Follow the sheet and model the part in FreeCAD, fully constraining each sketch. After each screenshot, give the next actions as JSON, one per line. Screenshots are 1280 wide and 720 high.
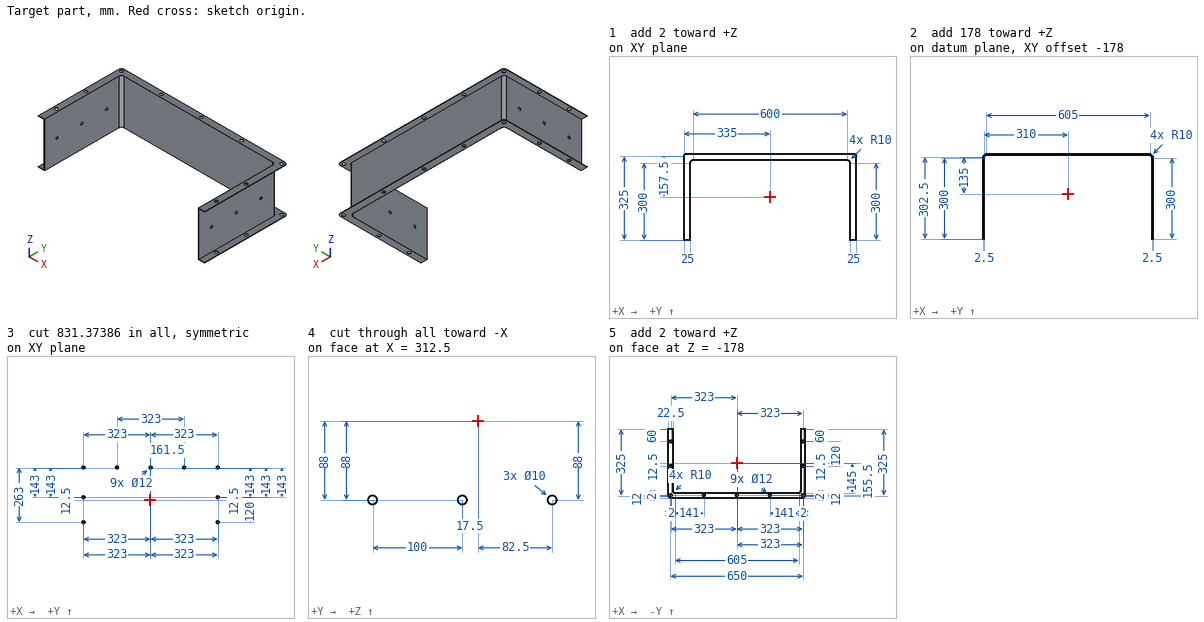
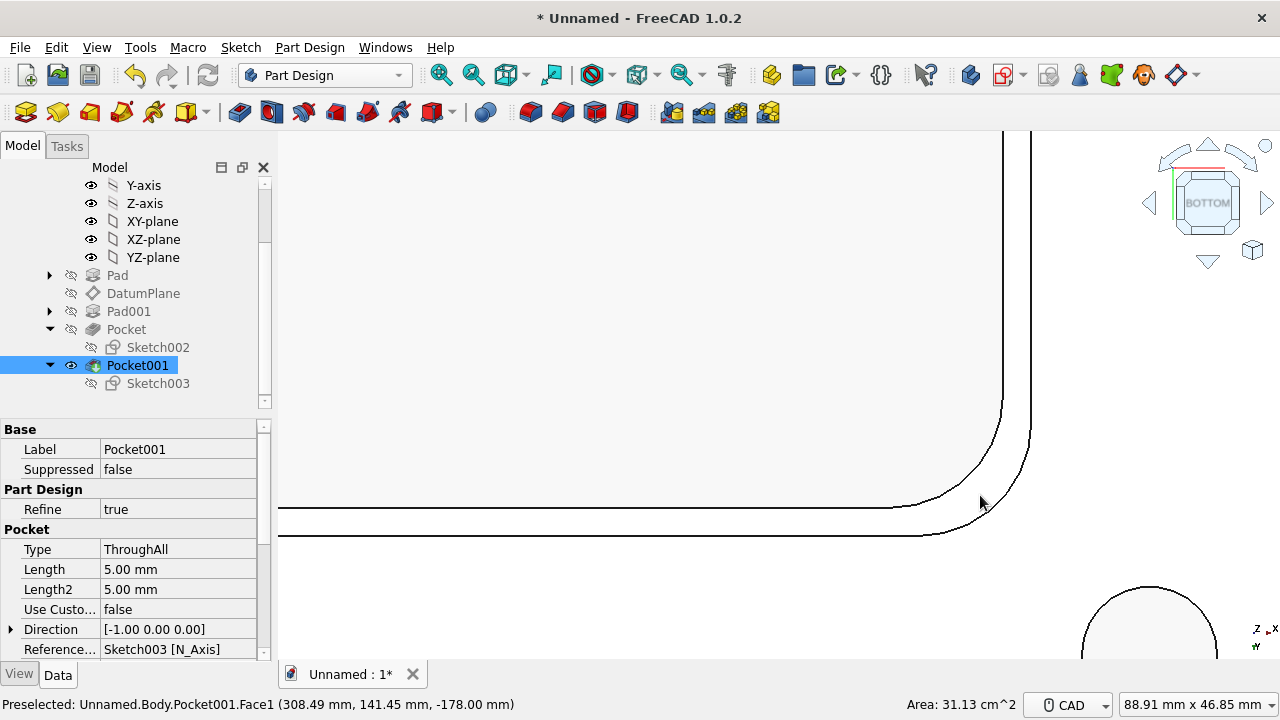
{"action": "left_click", "coordinate": [1004, 76]}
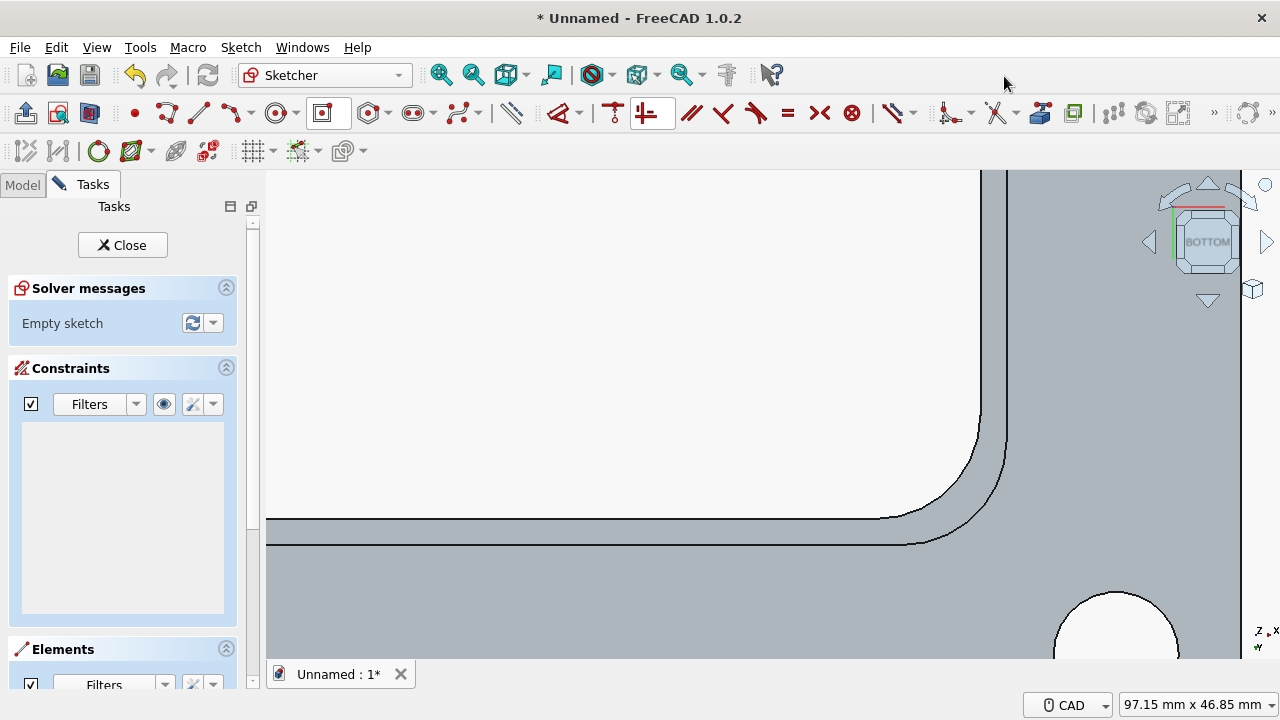
{"action": "scroll", "coordinate": [1000, 552], "scroll_direction": "down", "scroll_amount": 12}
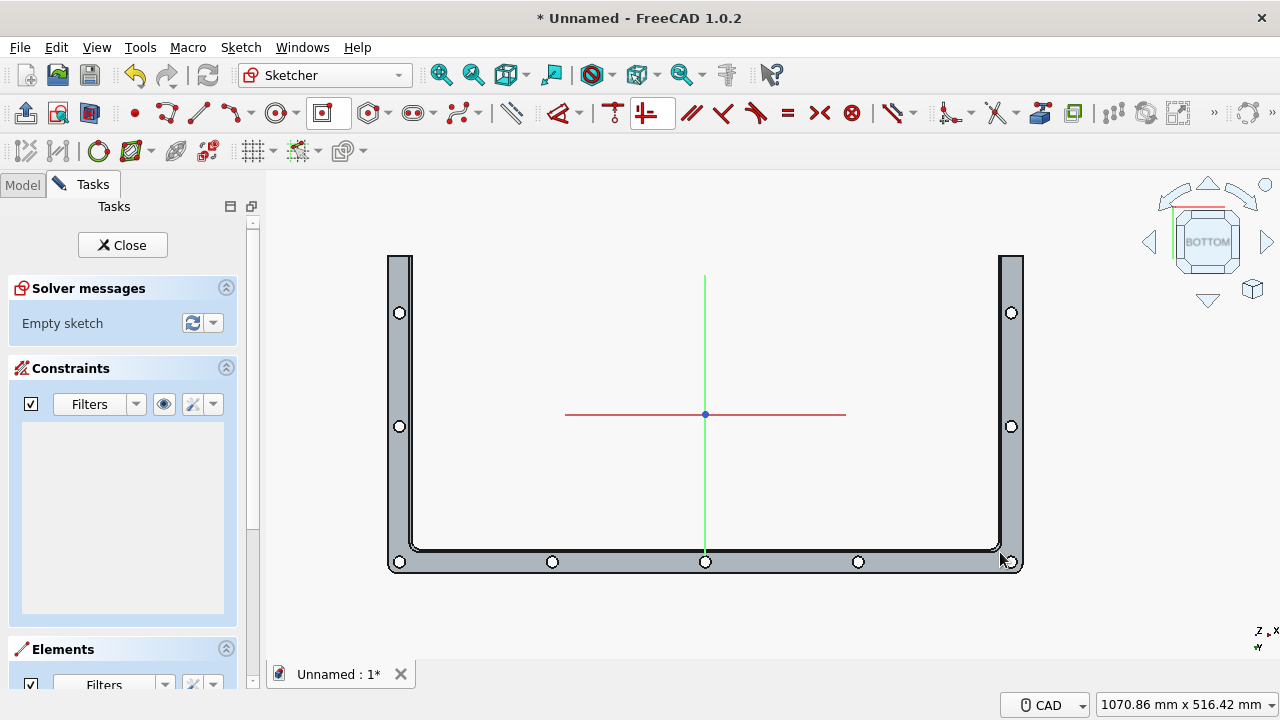
{"action": "left_click", "coordinate": [200, 114]}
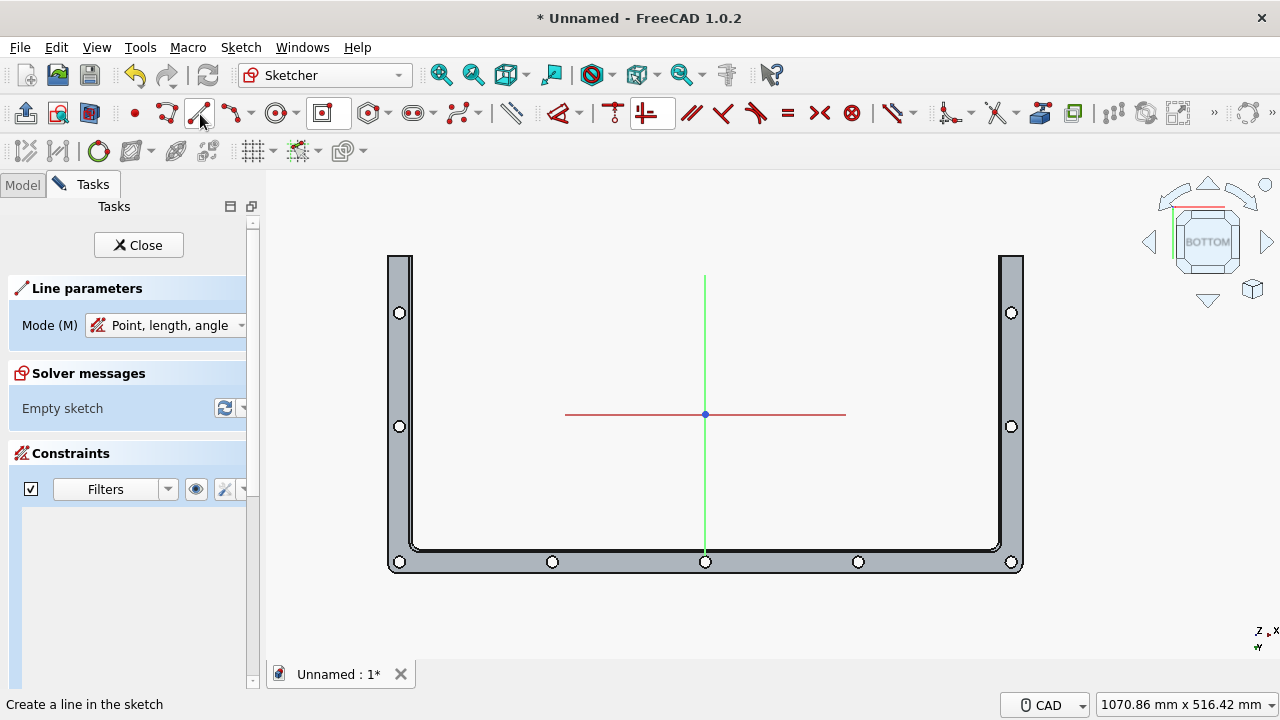
{"action": "left_click", "coordinate": [992, 552]}
{"action": "left_click", "coordinate": [419, 552]}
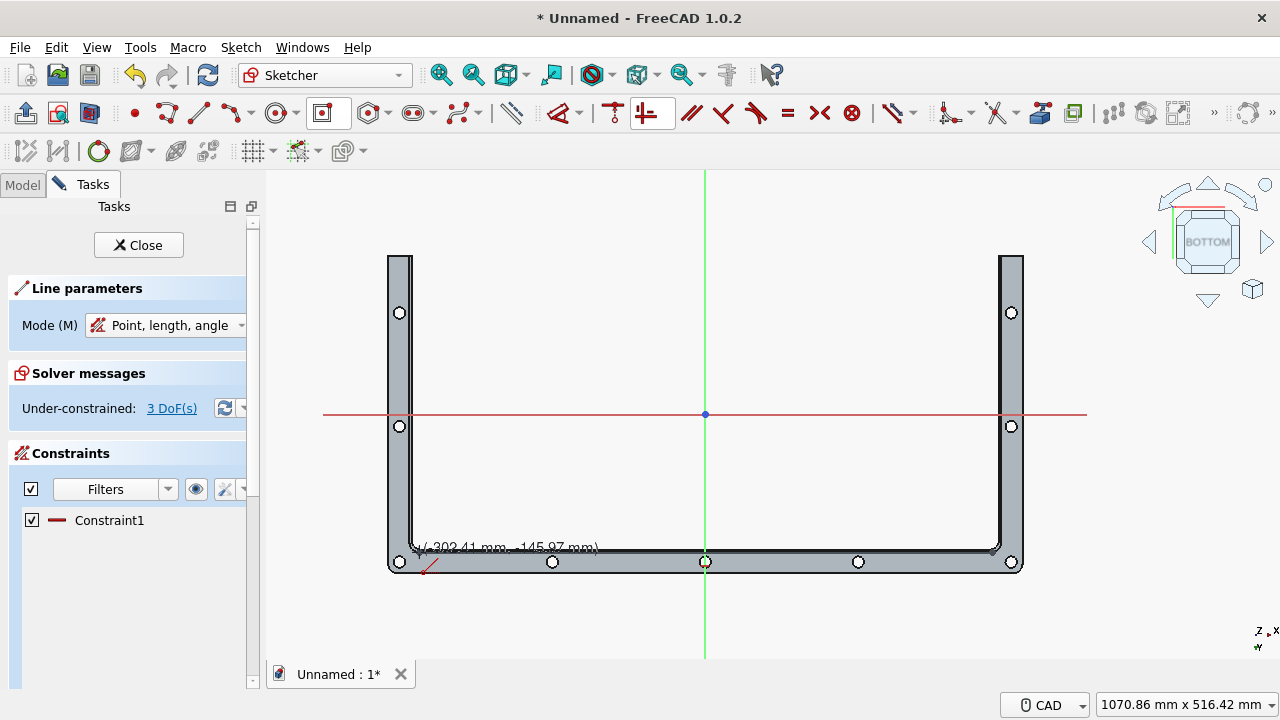
{"action": "key", "text": "g m"}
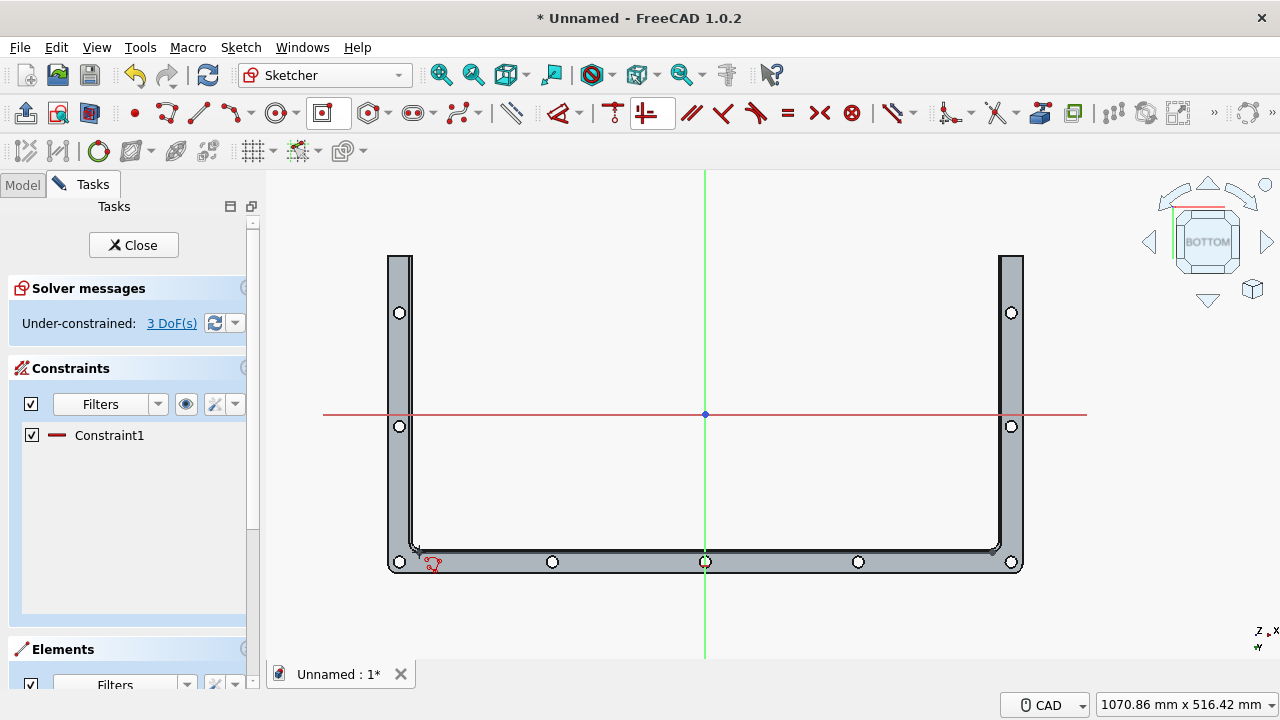
{"action": "left_click", "coordinate": [409, 543]}
{"action": "left_click", "coordinate": [409, 256]}
{"action": "left_click", "coordinate": [388, 256]}
{"action": "left_click", "coordinate": [388, 564]}
{"action": "right_click", "coordinate": [388, 564]}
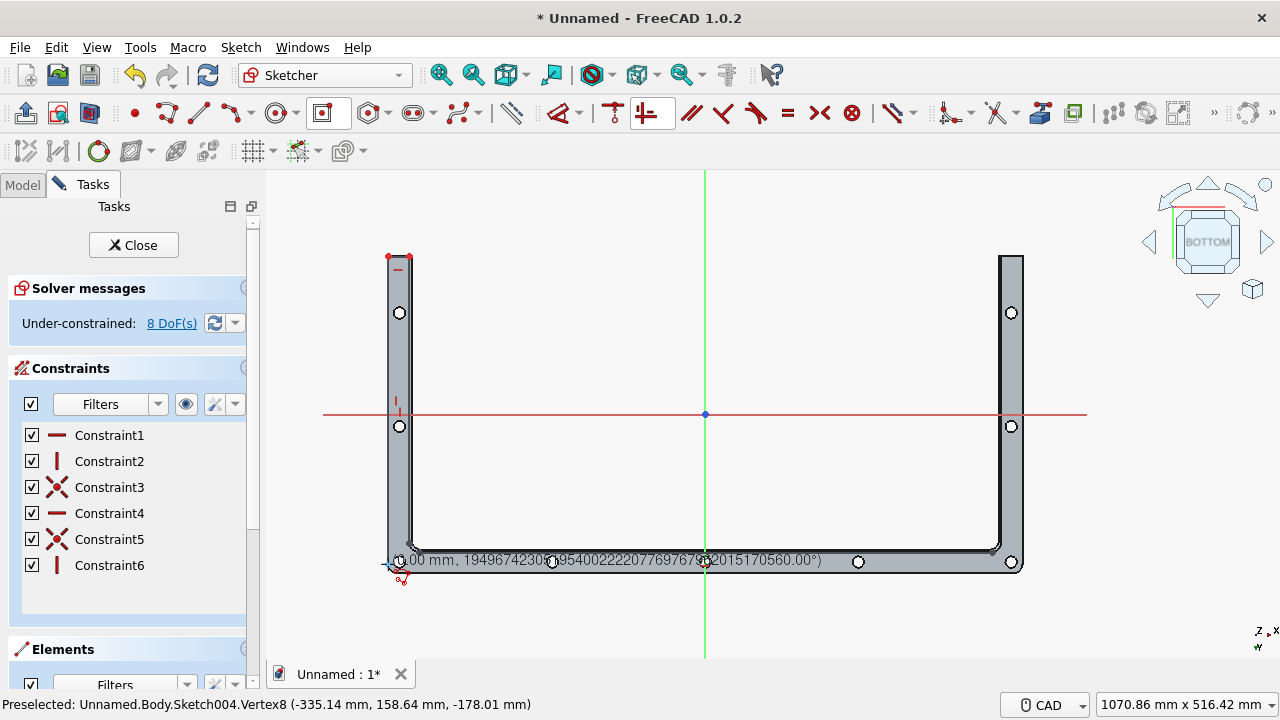
{"action": "left_click", "coordinate": [200, 114]}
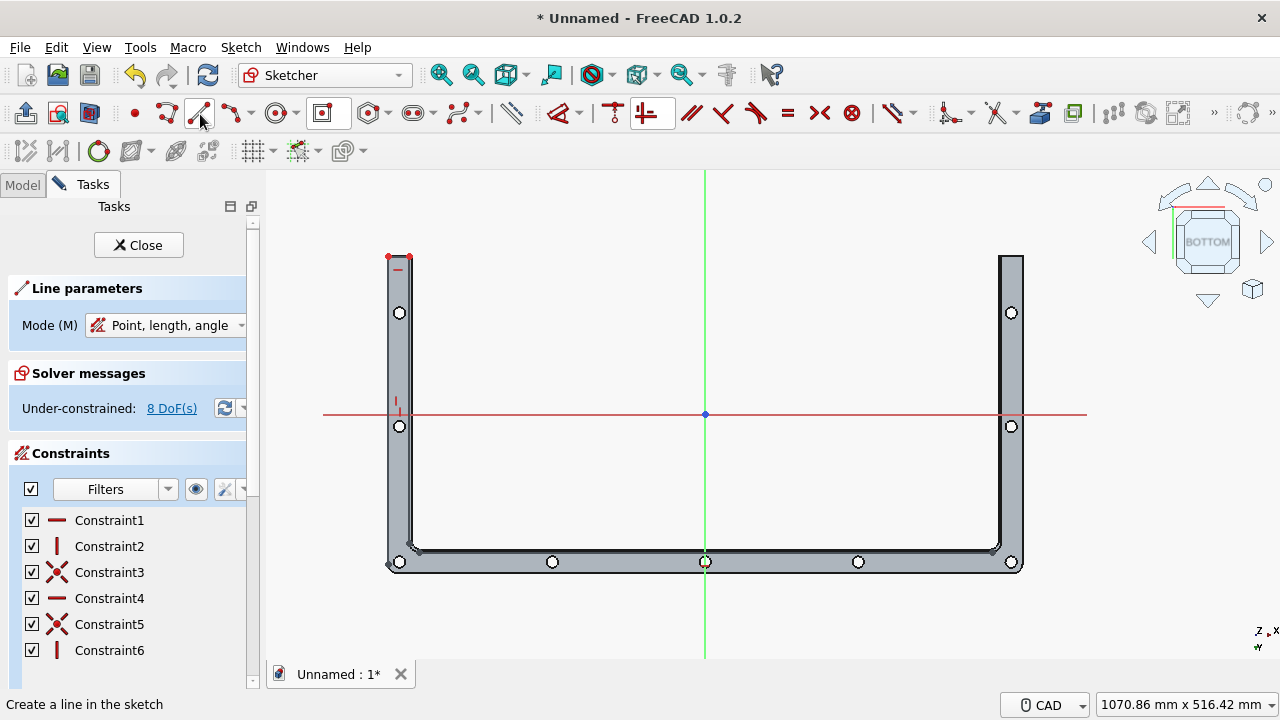
{"action": "left_click", "coordinate": [398, 573]}
{"action": "left_click", "coordinate": [1013, 573]}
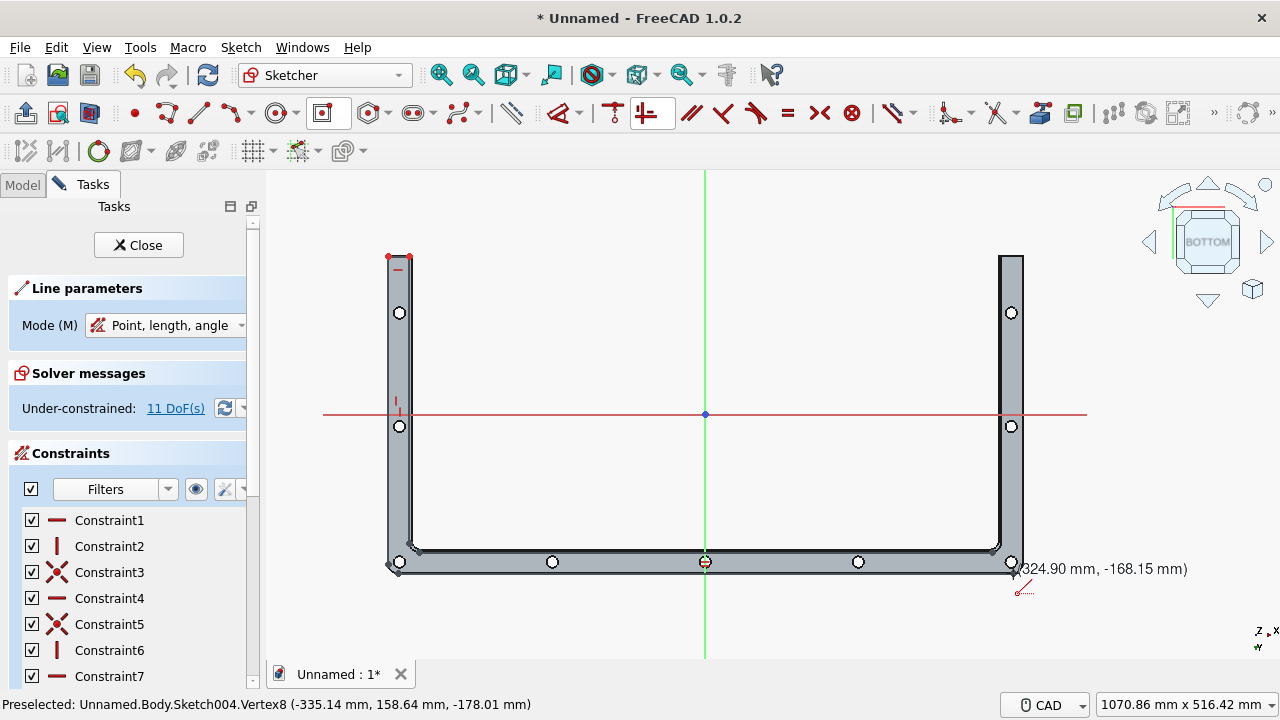
{"action": "left_click", "coordinate": [168, 114]}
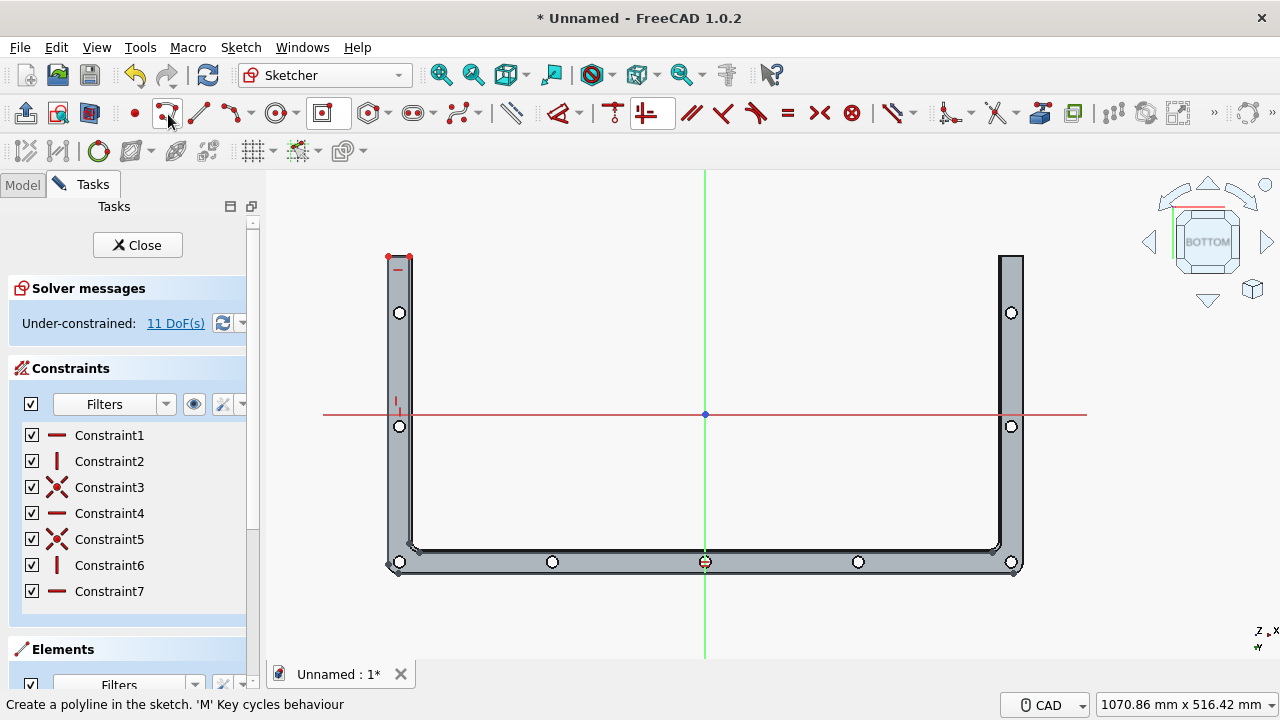
{"action": "left_click", "coordinate": [1023, 564]}
{"action": "left_click", "coordinate": [1023, 256]}
{"action": "left_click", "coordinate": [1001, 256]}
{"action": "left_click", "coordinate": [1001, 543]}
{"action": "right_click", "coordinate": [1001, 543]}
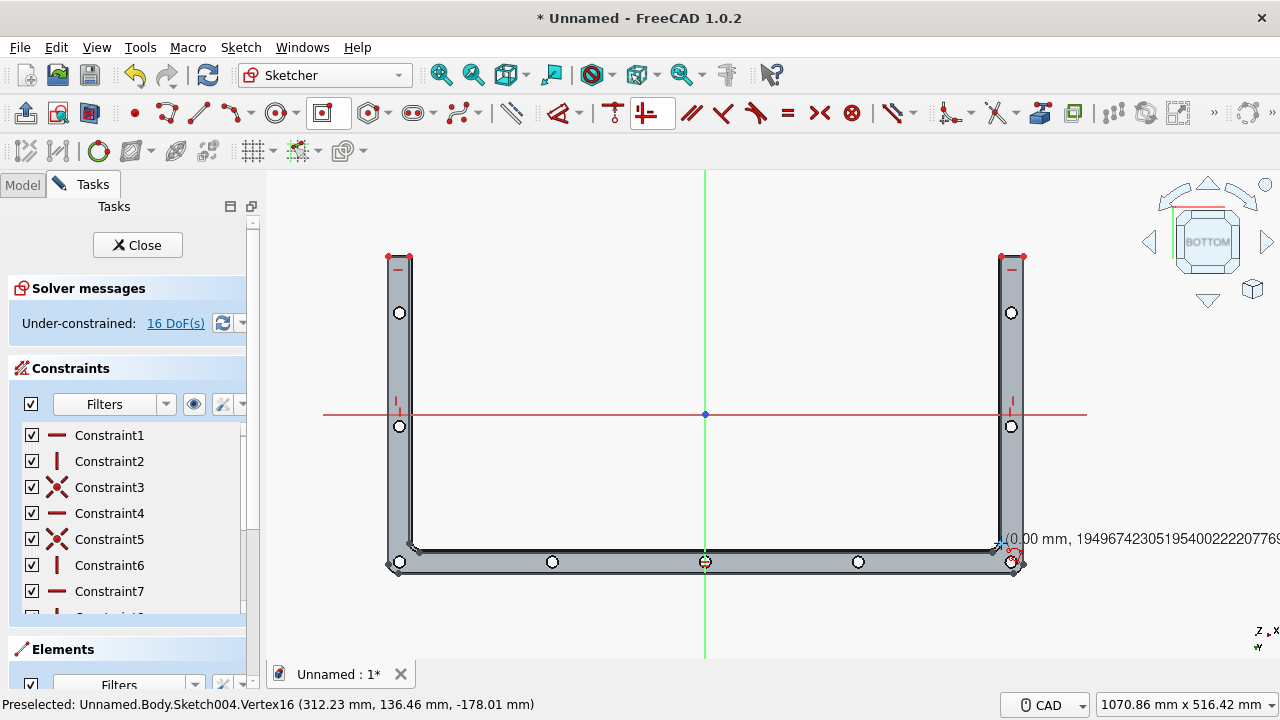
{"action": "key", "text": "g 3 a"}